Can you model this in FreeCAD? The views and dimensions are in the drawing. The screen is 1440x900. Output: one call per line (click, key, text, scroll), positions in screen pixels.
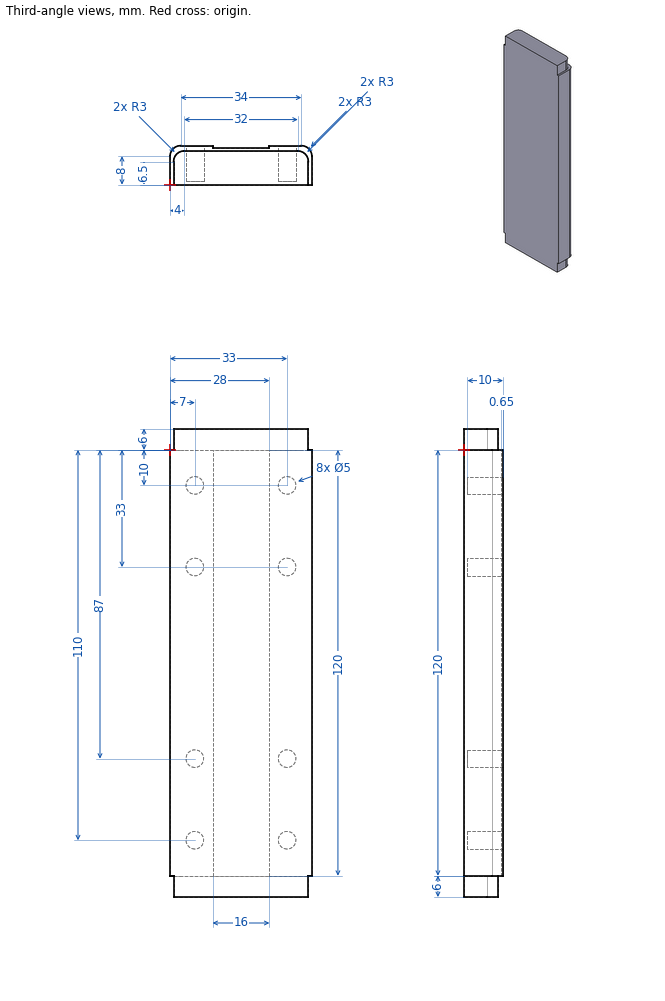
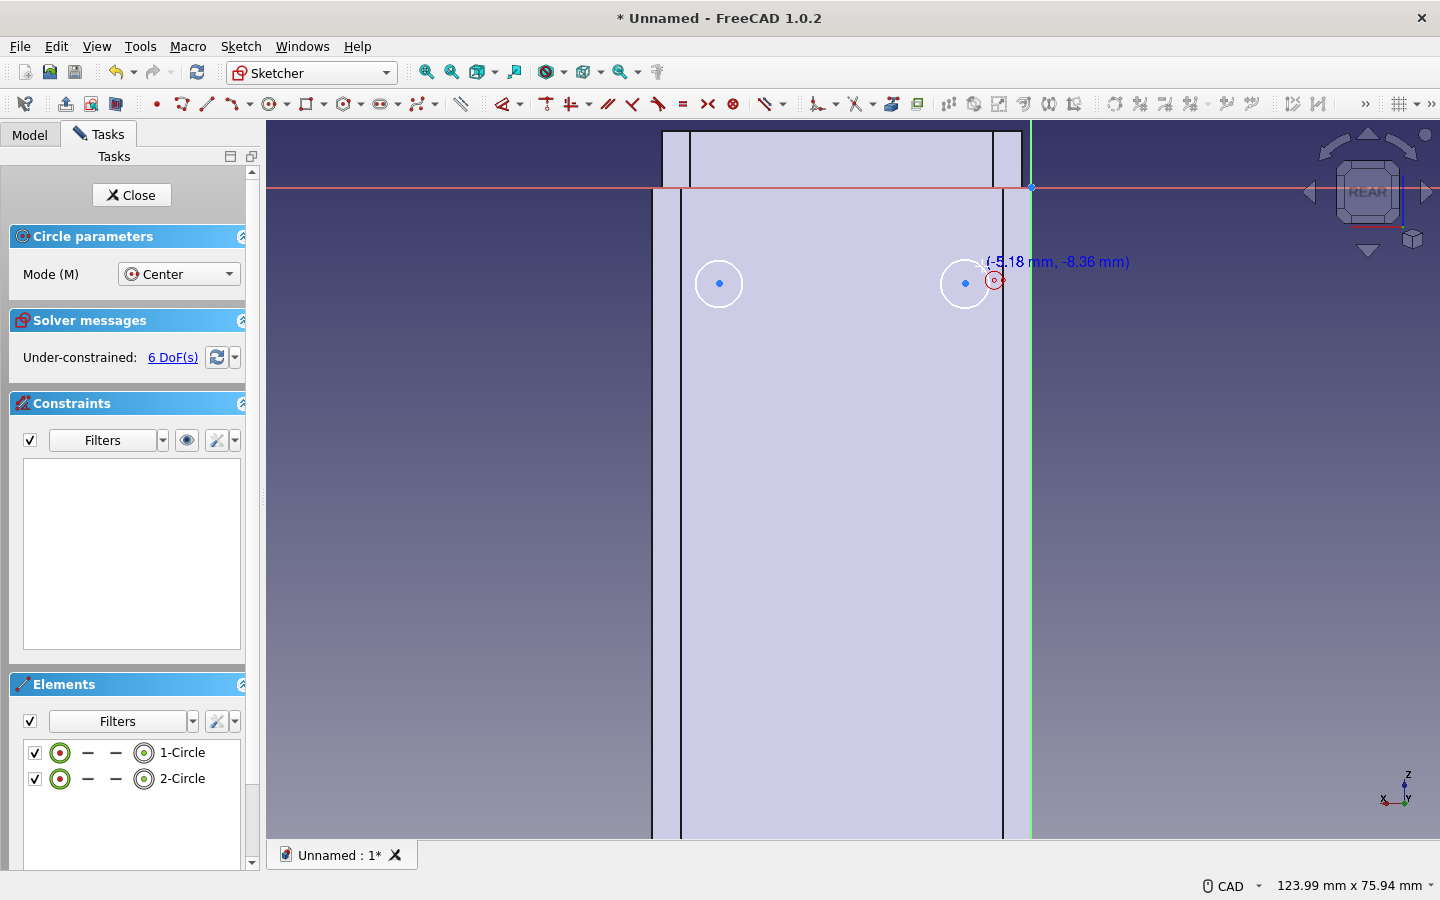
click(719, 500)
click(735, 484)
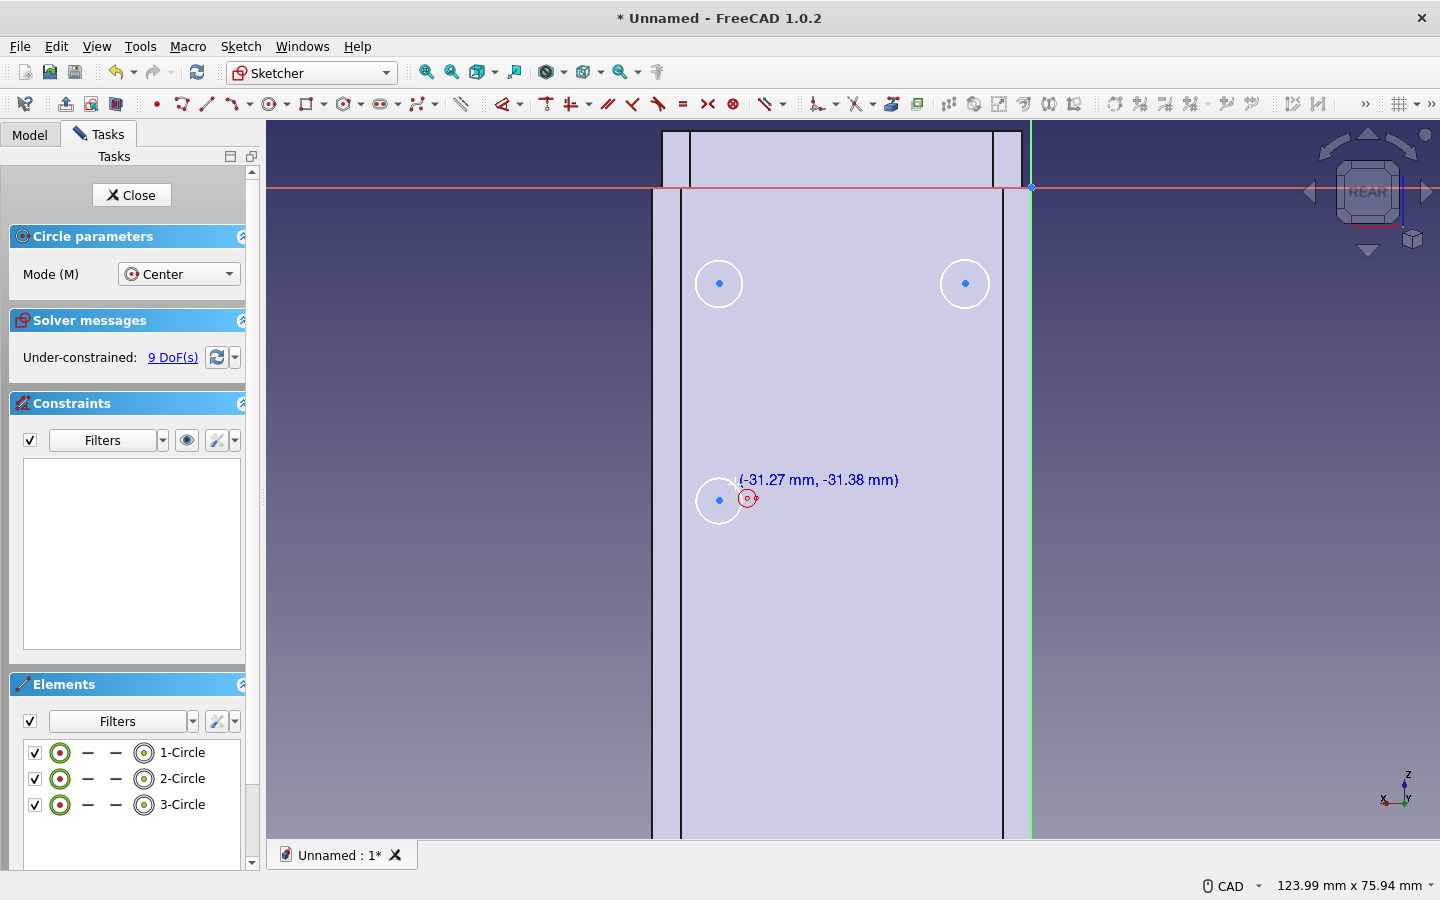
click(965, 500)
click(982, 484)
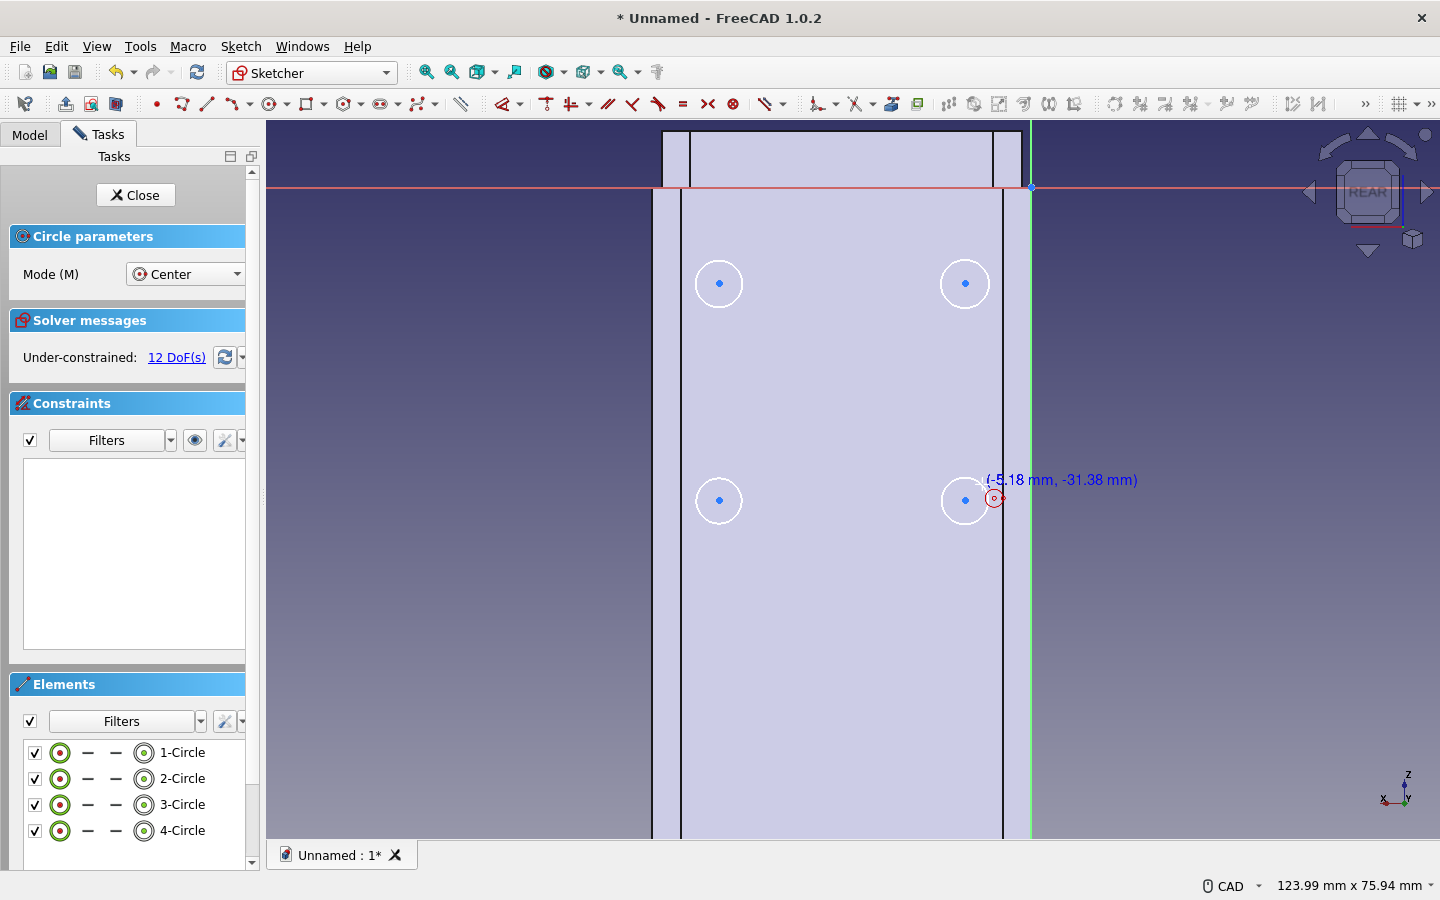
scroll(720, 283, down, 4)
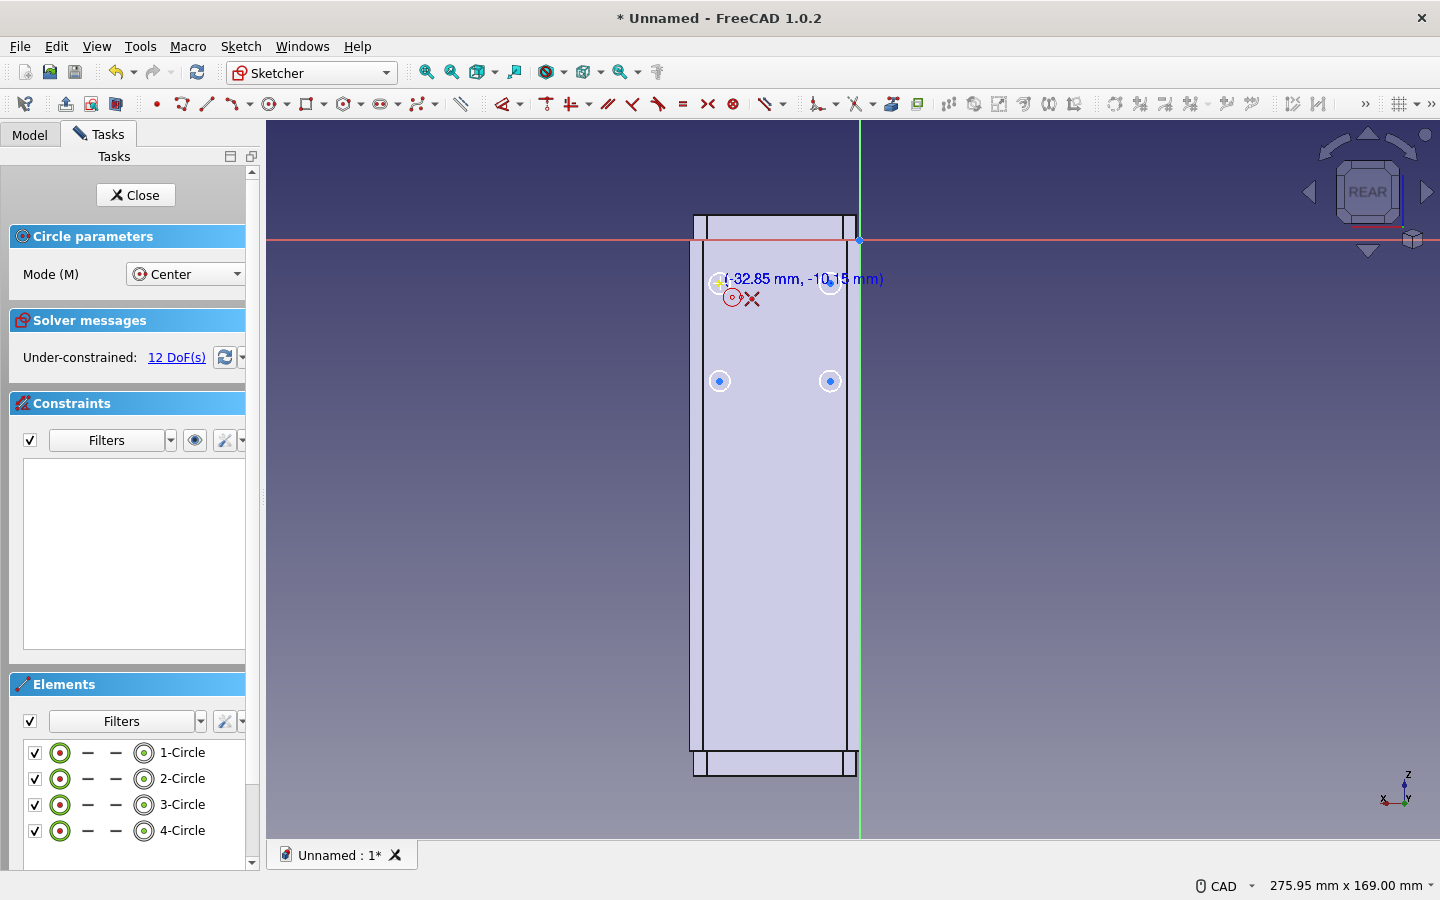
scroll(830, 611, up, 4)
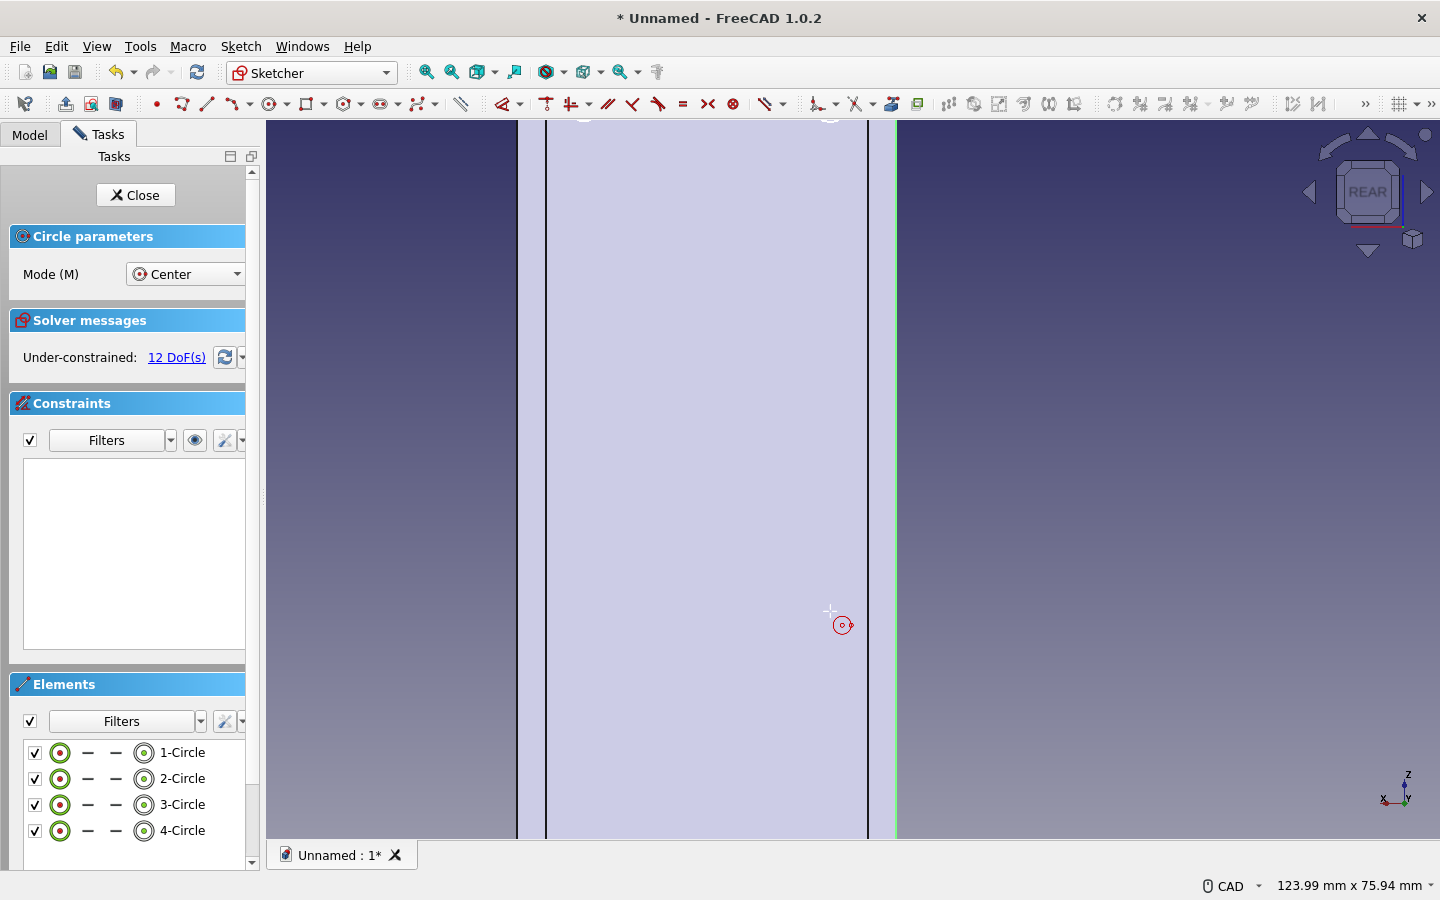
click(830, 609)
click(847, 592)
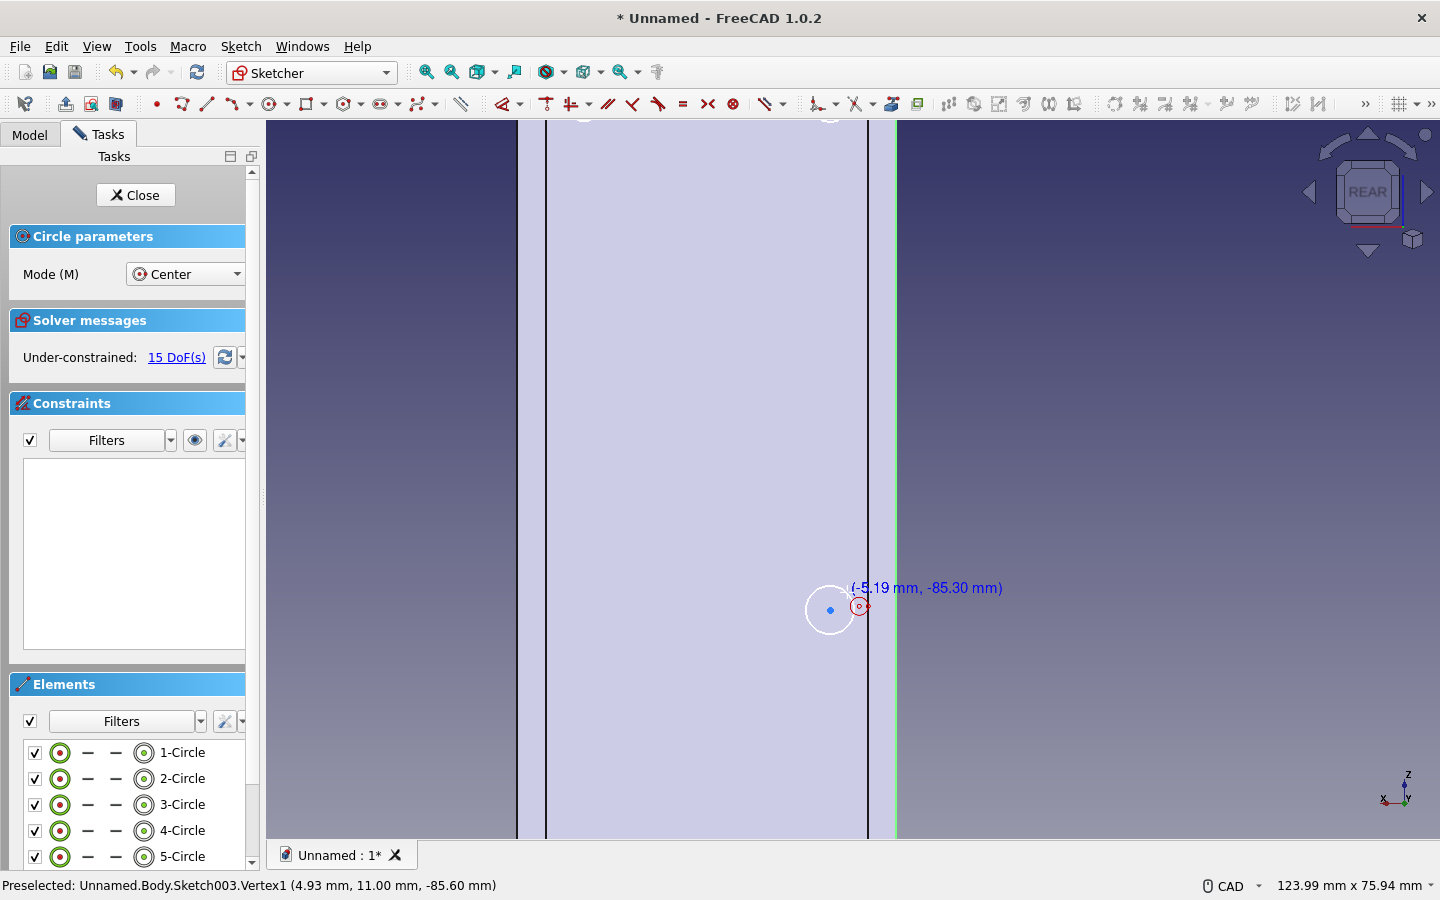
click(584, 609)
click(600, 592)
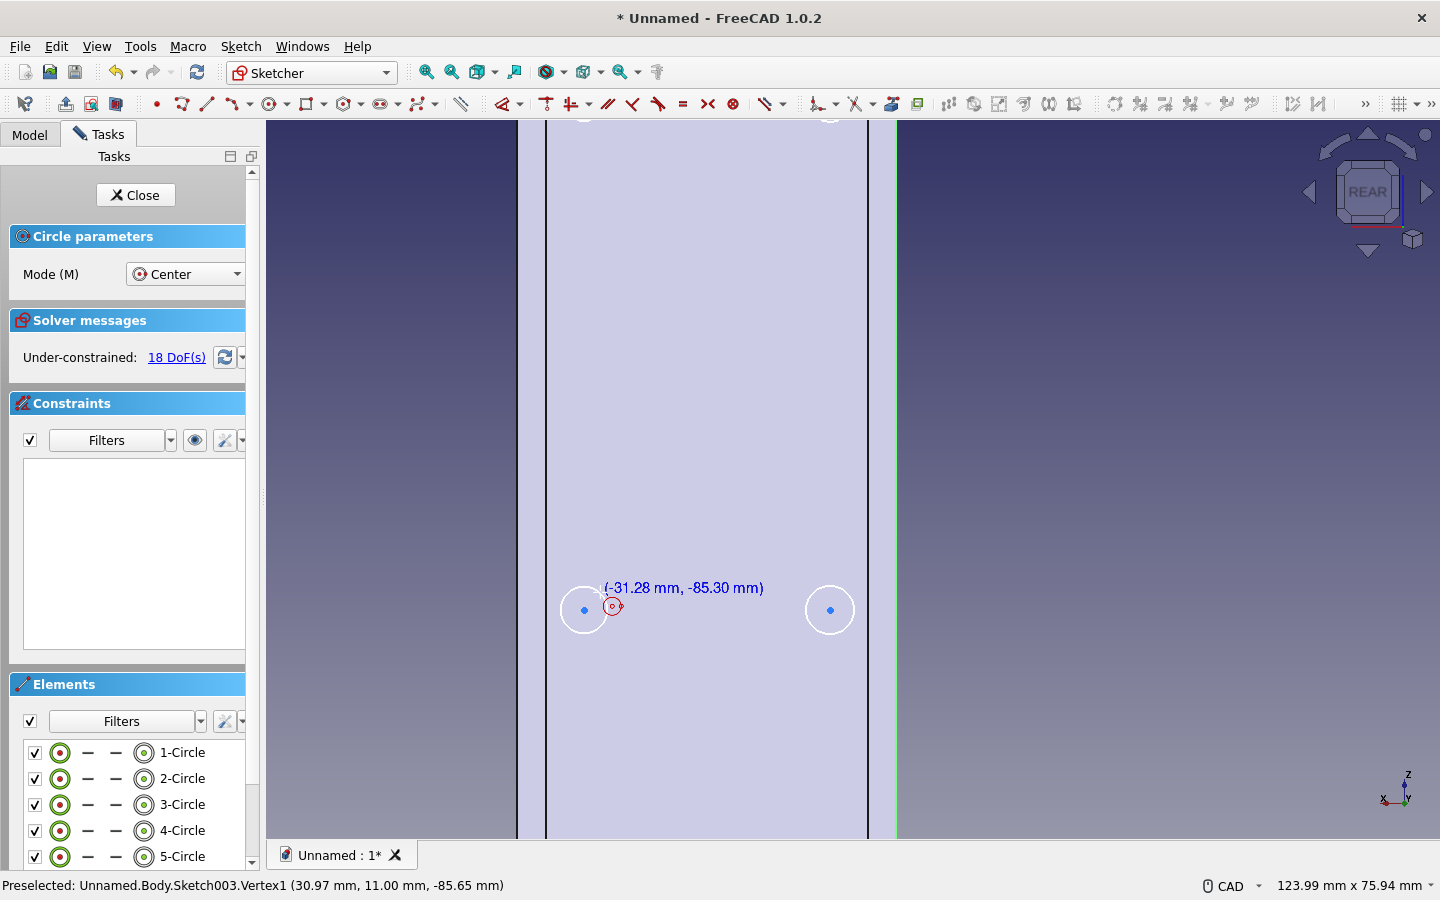
scroll(831, 611, down, 4)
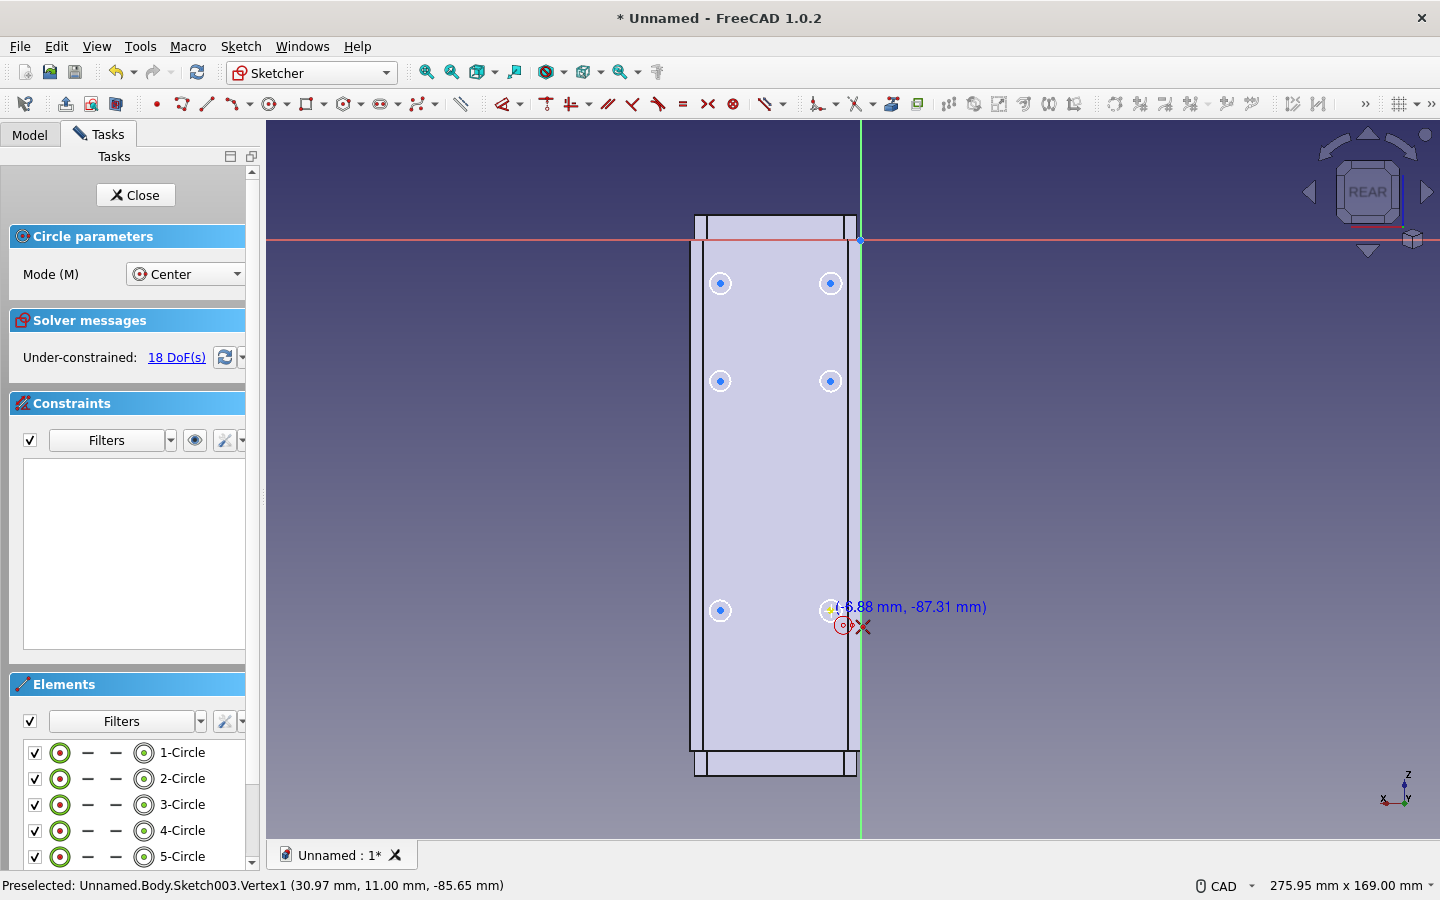
scroll(831, 708, up, 4)